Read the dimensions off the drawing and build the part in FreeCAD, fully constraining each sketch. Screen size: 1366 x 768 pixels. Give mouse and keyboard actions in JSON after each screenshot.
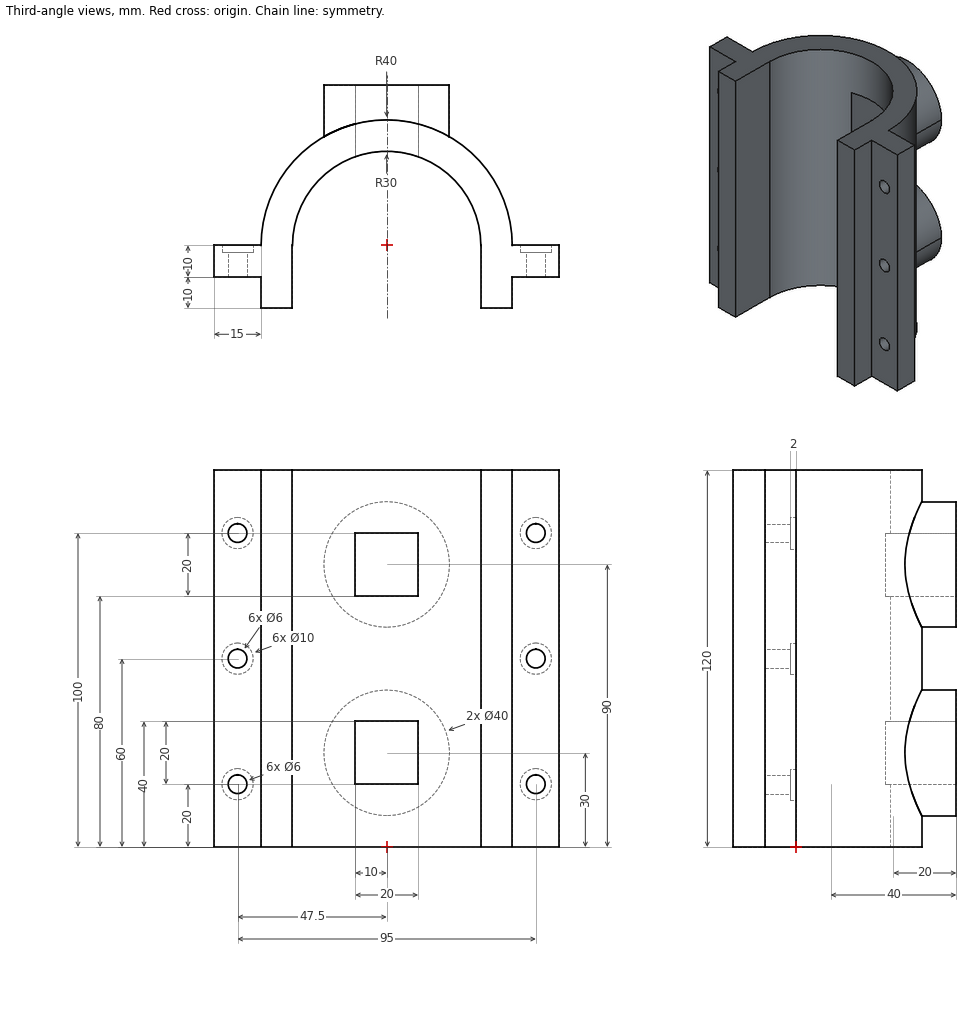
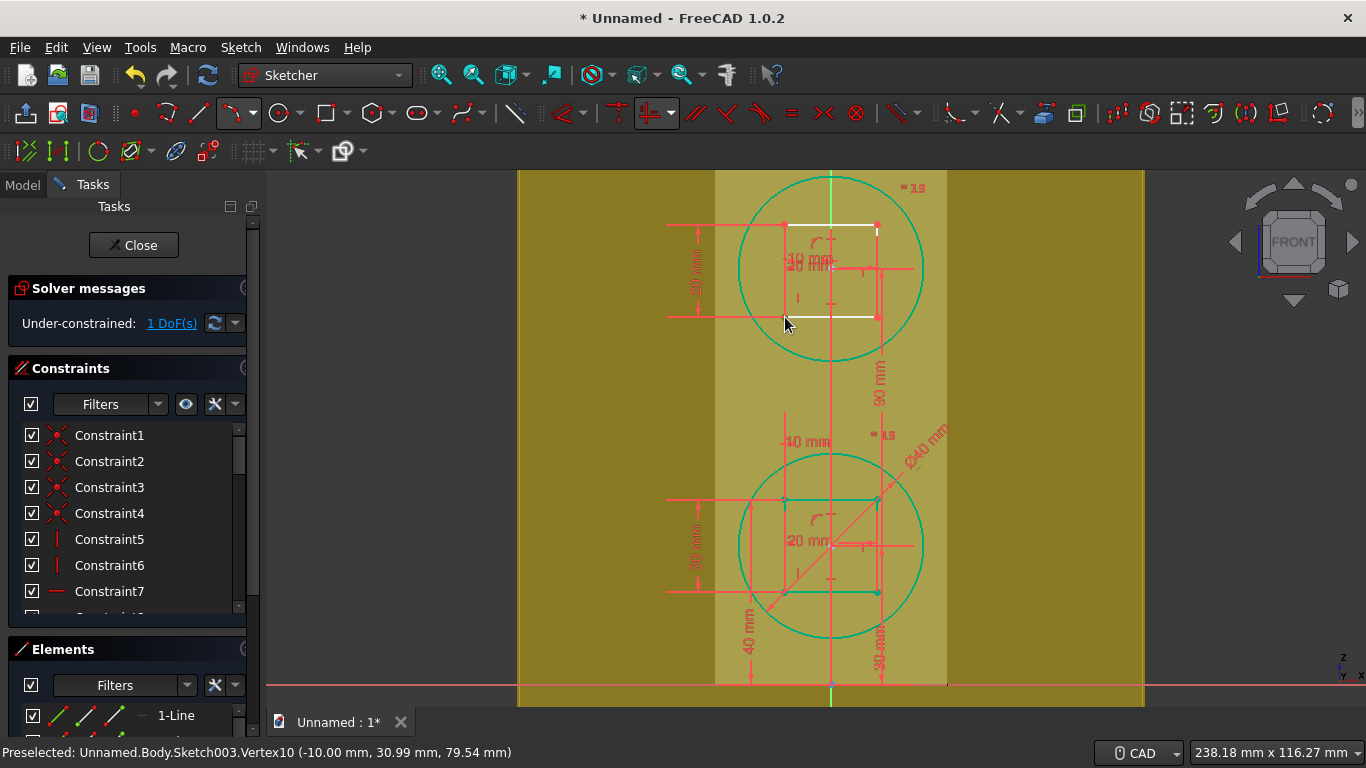
{"action": "key", "text": "i"}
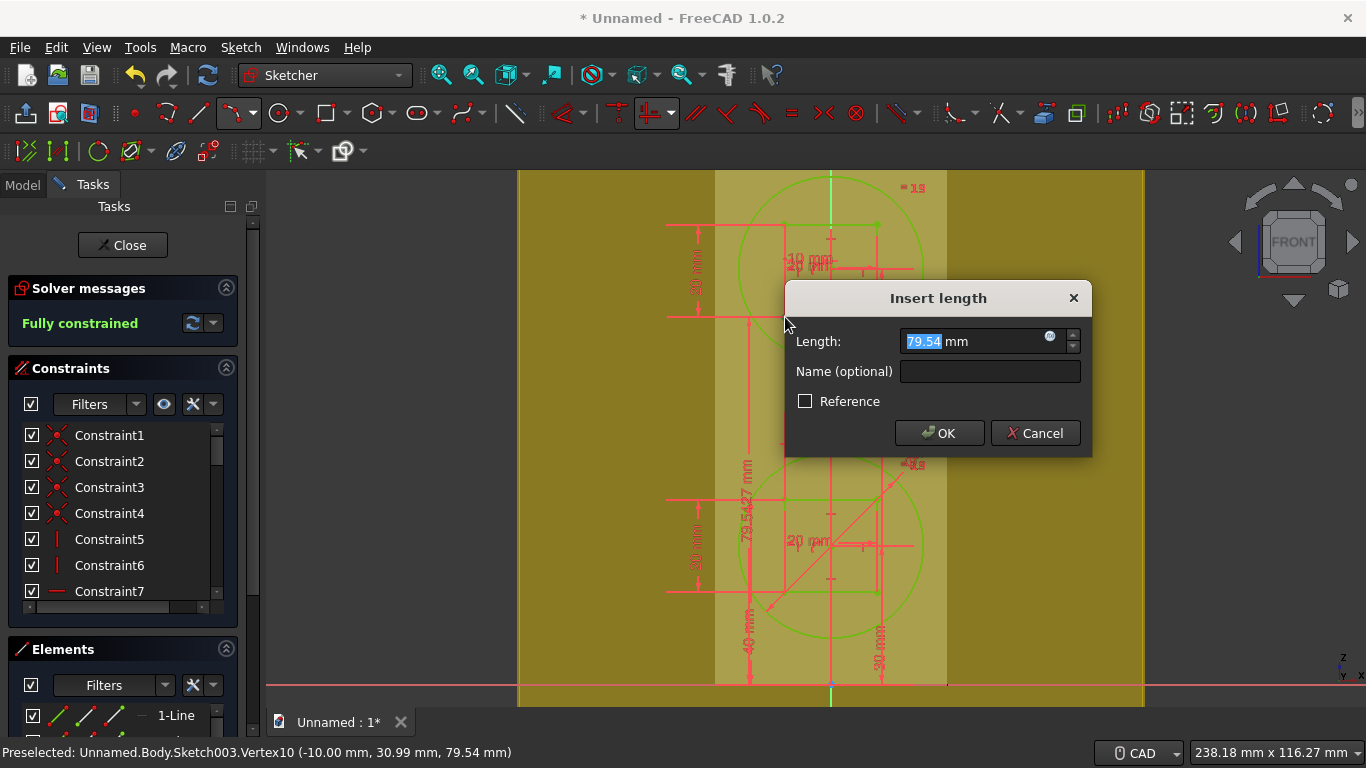
{"action": "type", "text": "80"}
{"action": "key", "text": "Return"}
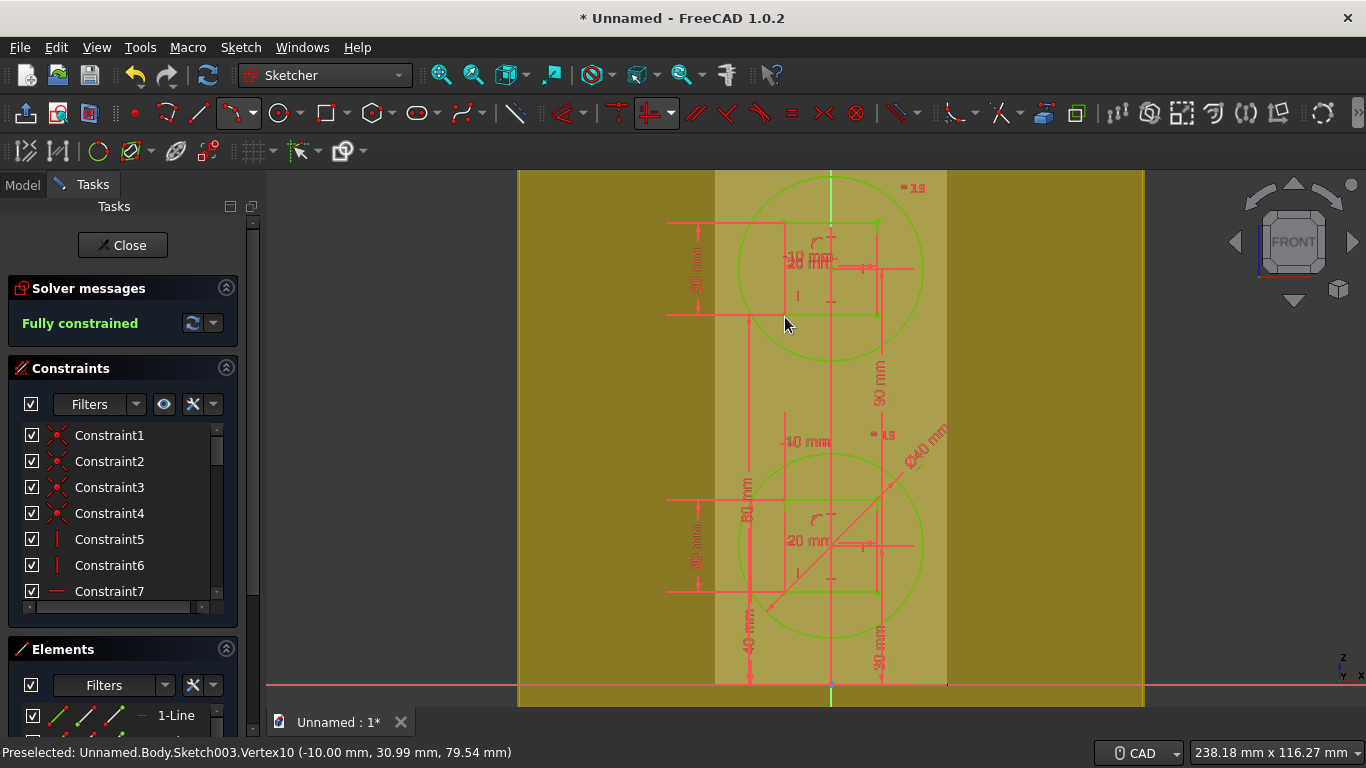
{"action": "left_click", "coordinate": [123, 245]}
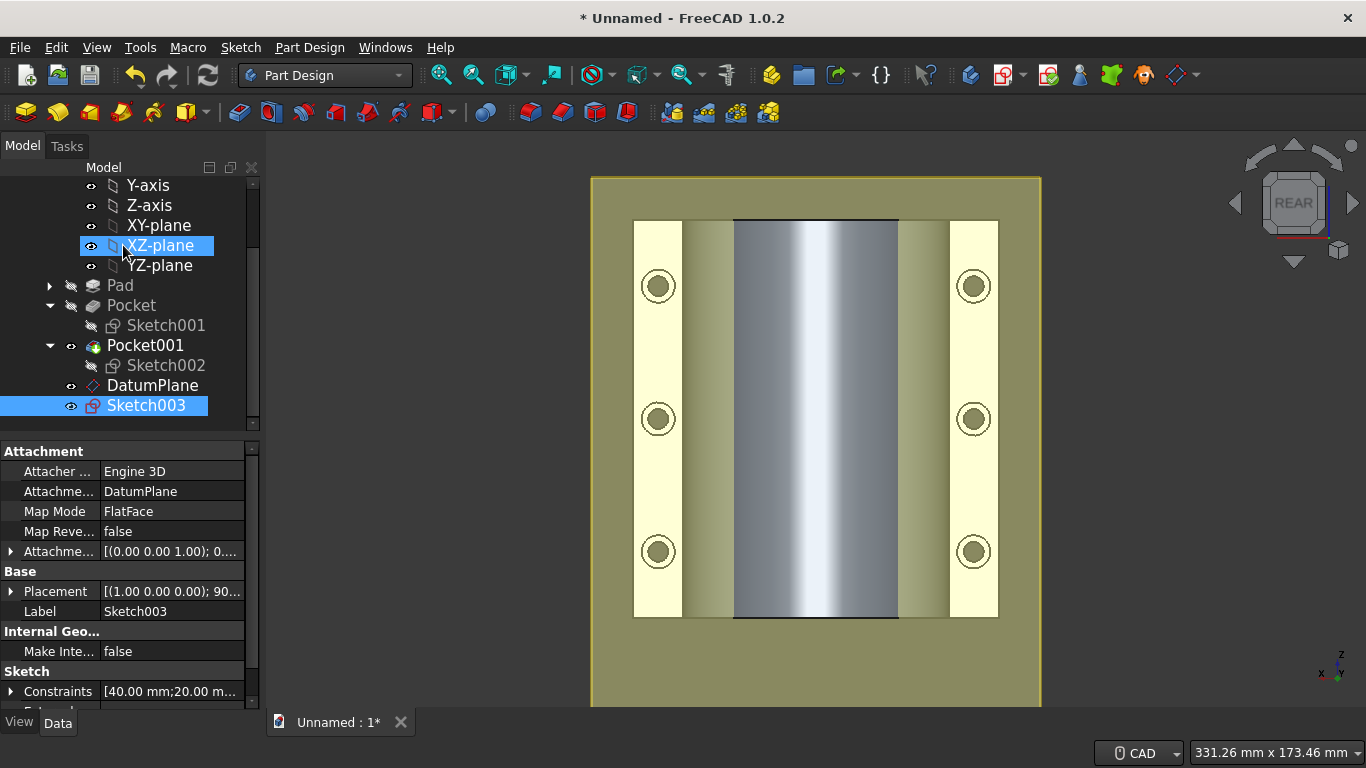
{"action": "left_click", "coordinate": [26, 112]}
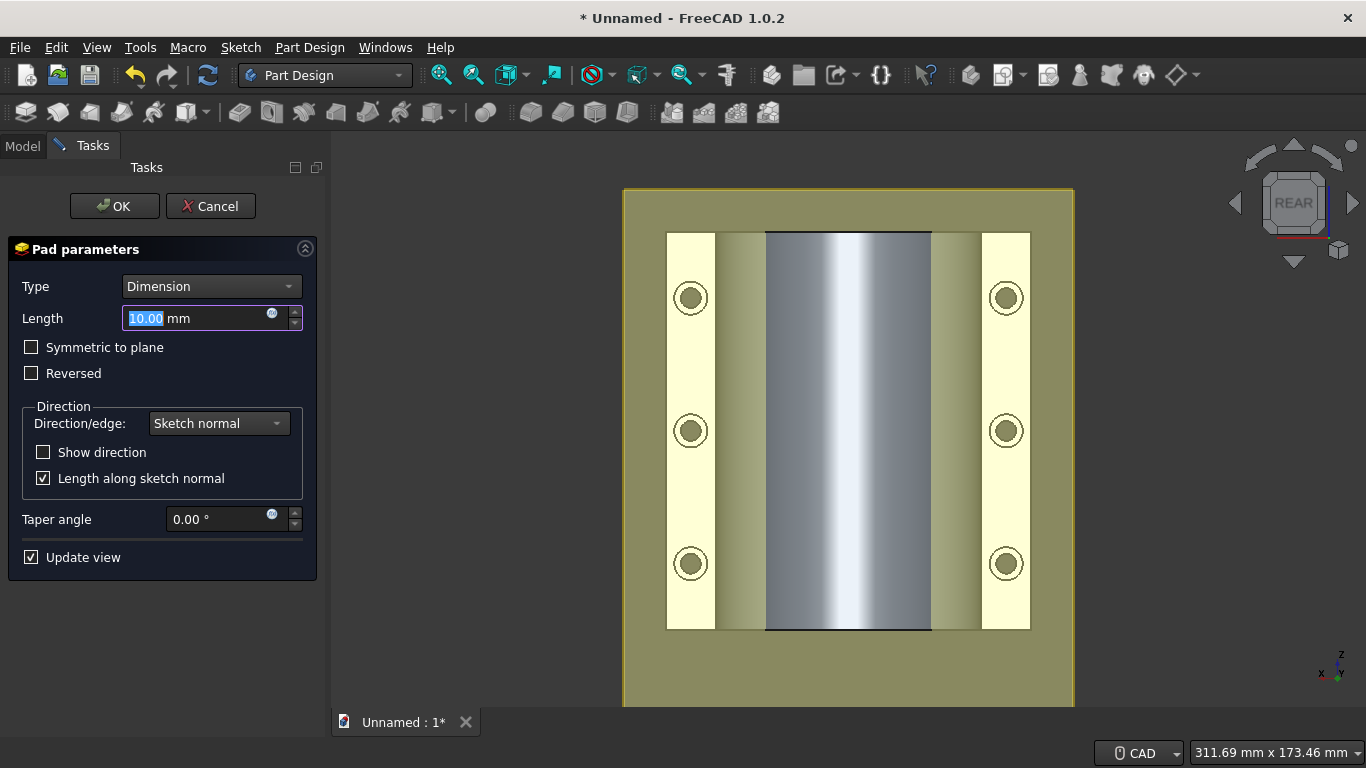
{"action": "type", "text": "20"}
{"action": "key", "text": "Tab"}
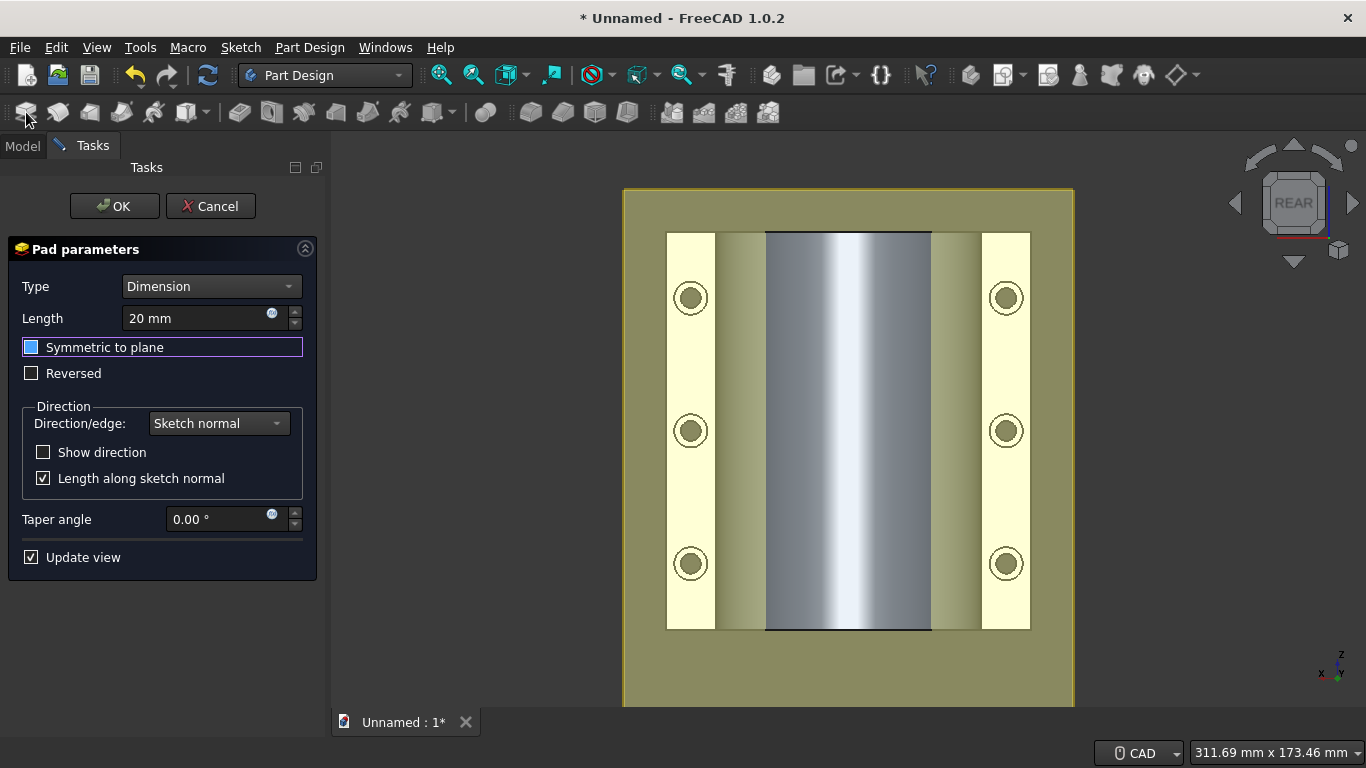
{"action": "left_click", "coordinate": [30, 373]}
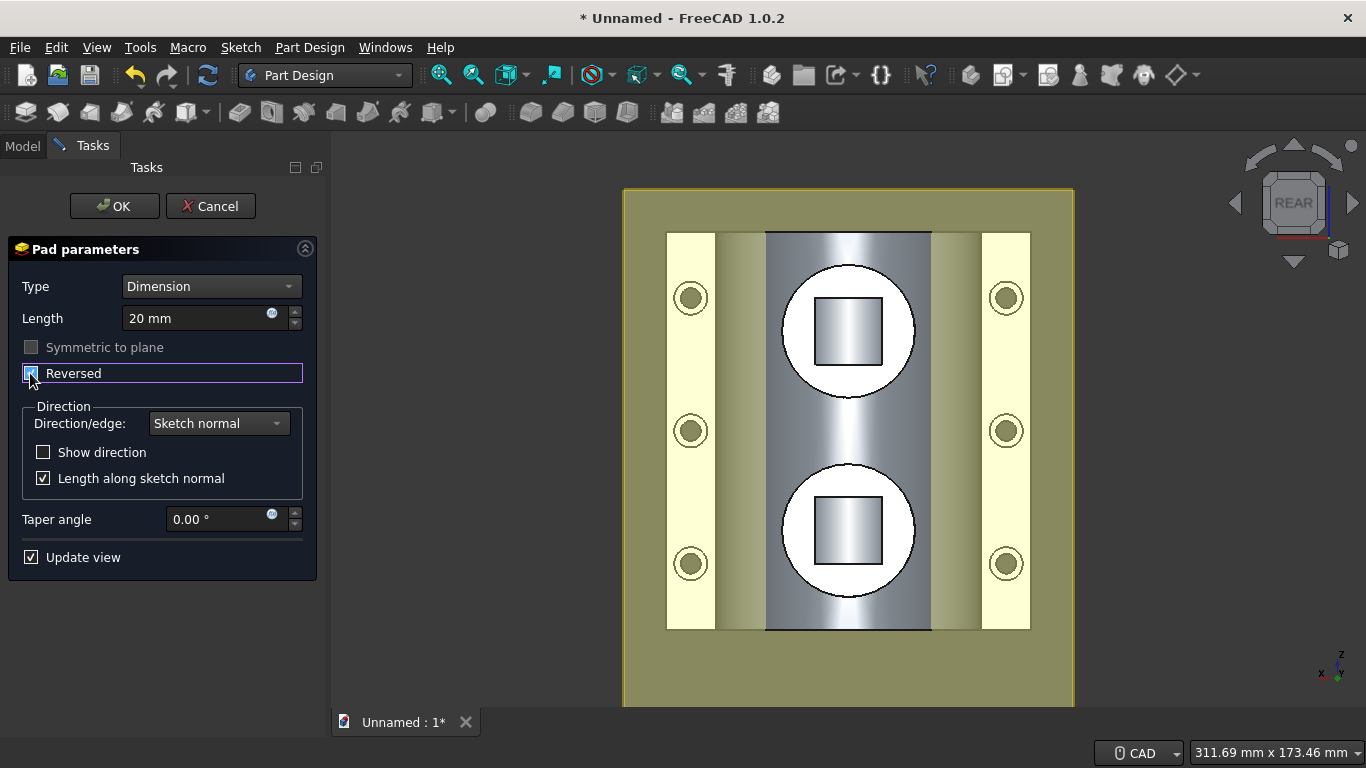
{"action": "left_click", "coordinate": [115, 206]}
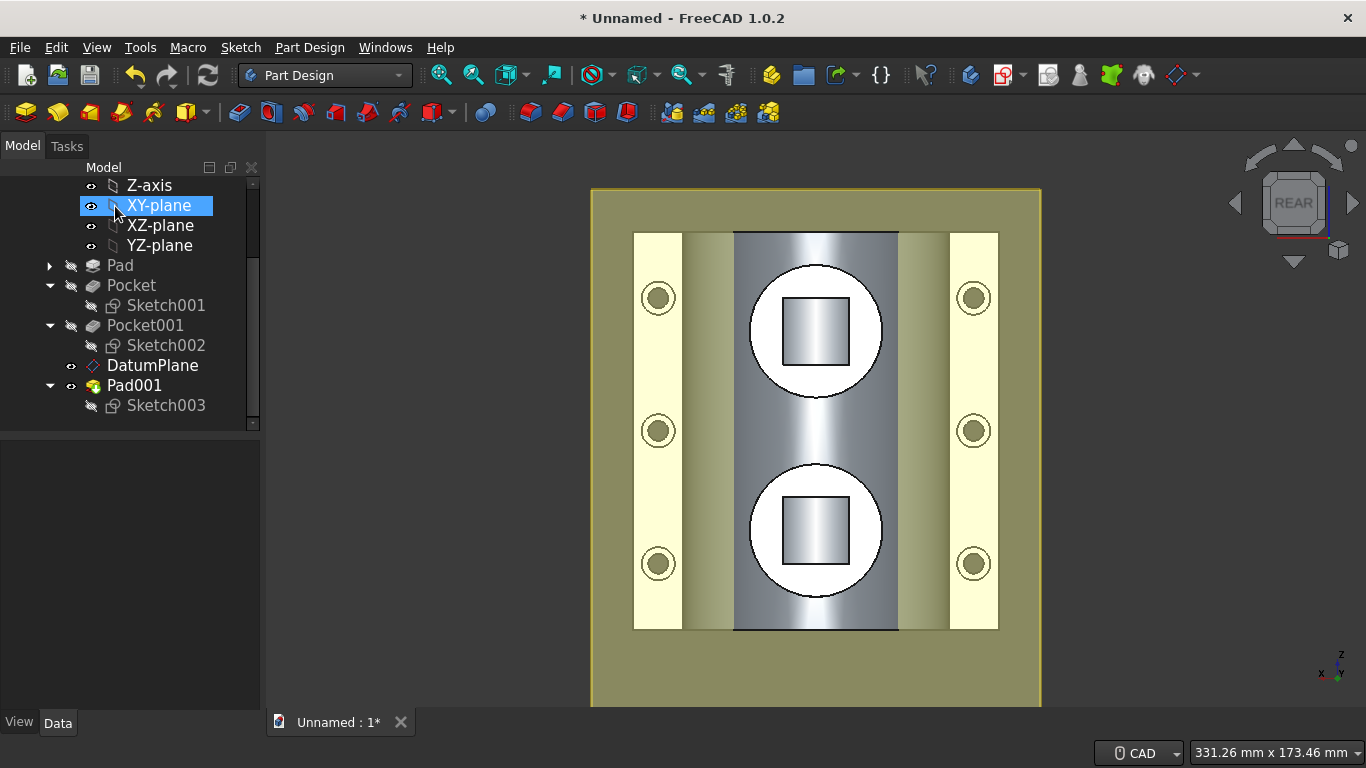
{"action": "left_click", "coordinate": [116, 366]}
{"action": "key", "text": "space"}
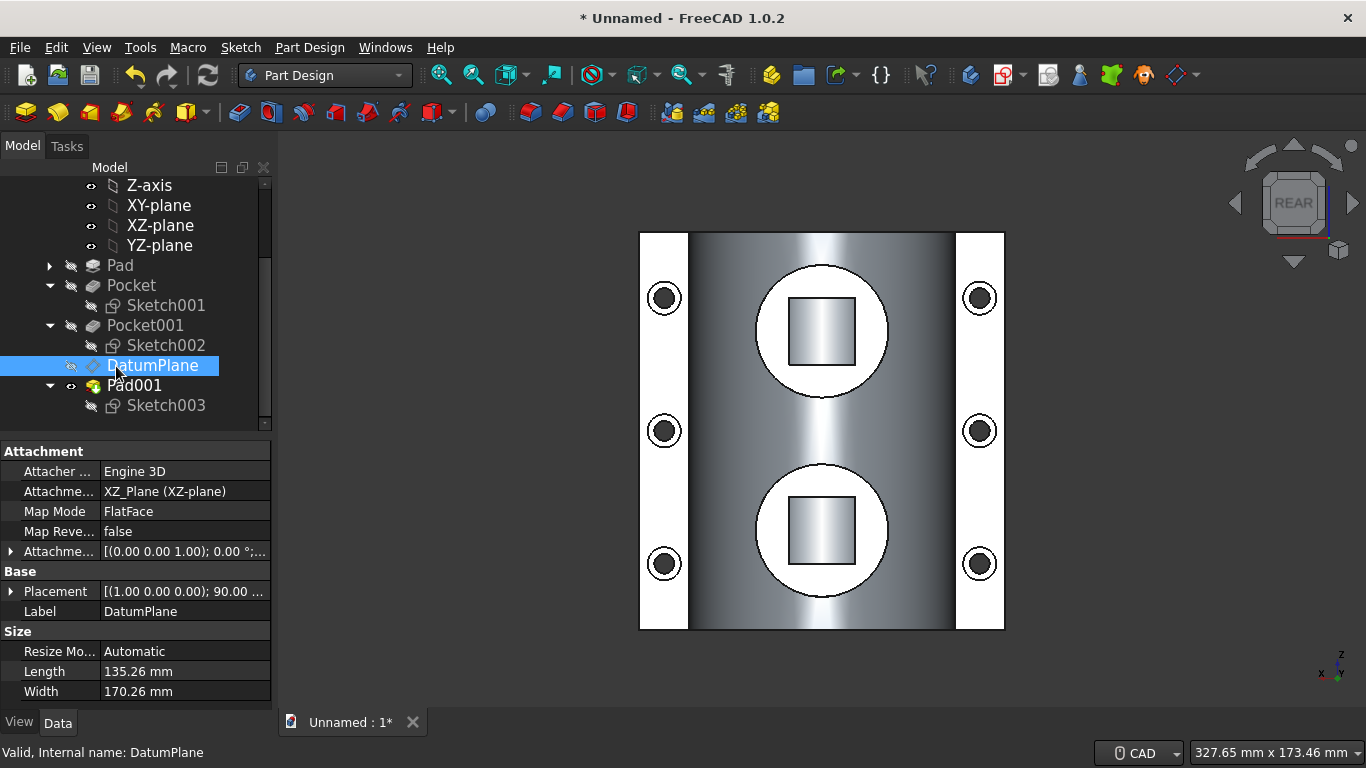
{"action": "scroll", "coordinate": [160, 301], "scroll_direction": "down", "scroll_amount": 3}